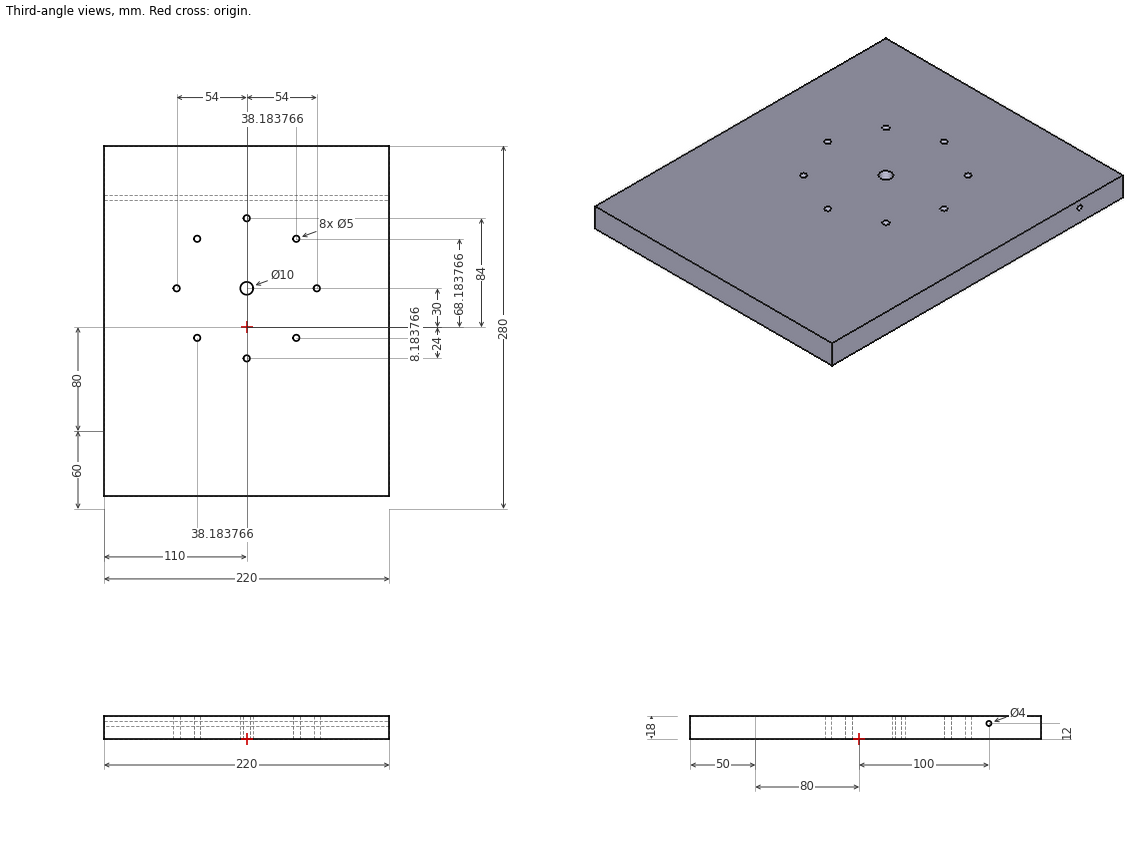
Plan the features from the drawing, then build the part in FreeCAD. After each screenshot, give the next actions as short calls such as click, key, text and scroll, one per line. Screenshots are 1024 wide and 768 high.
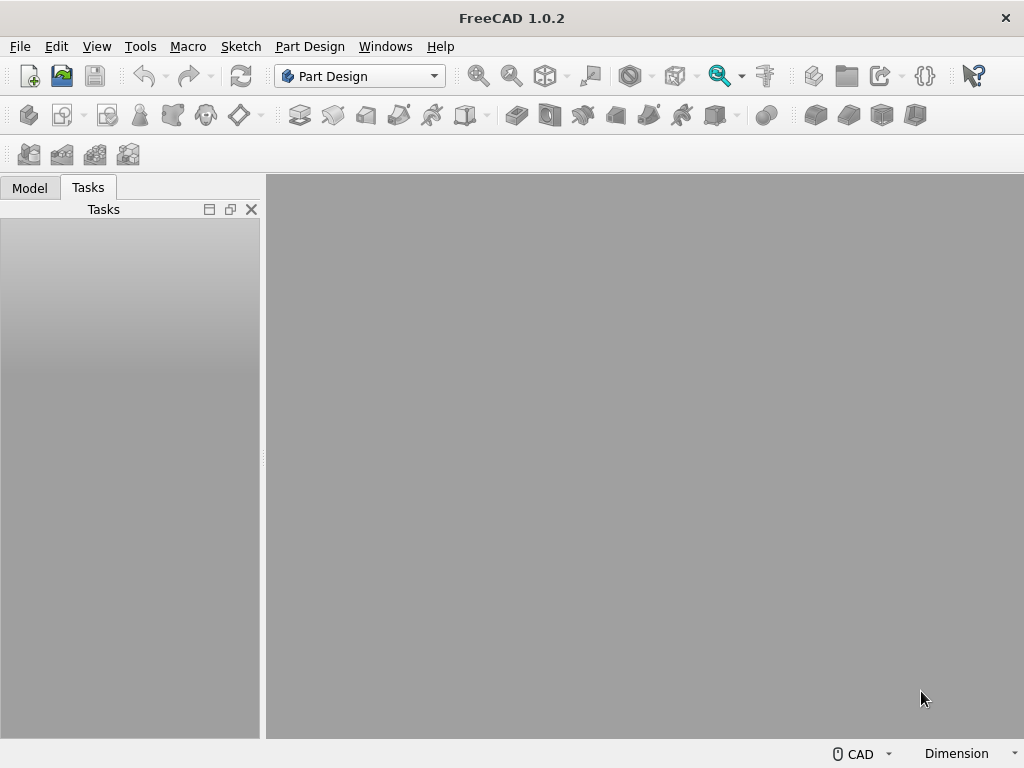
click(29, 76)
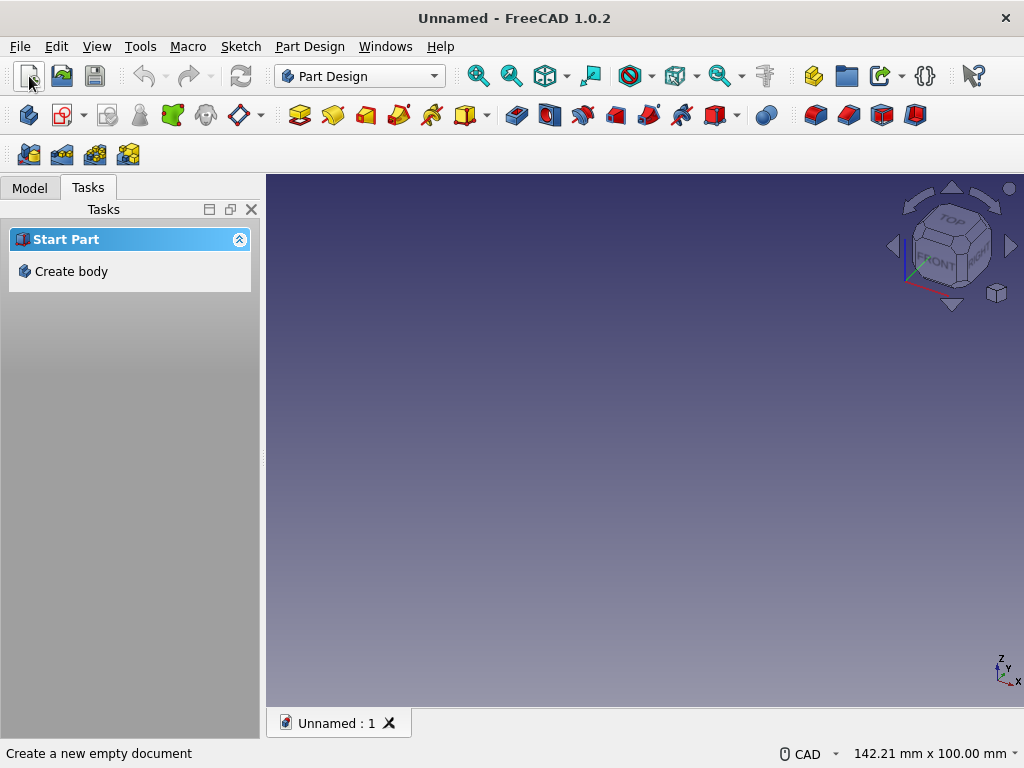
click(62, 116)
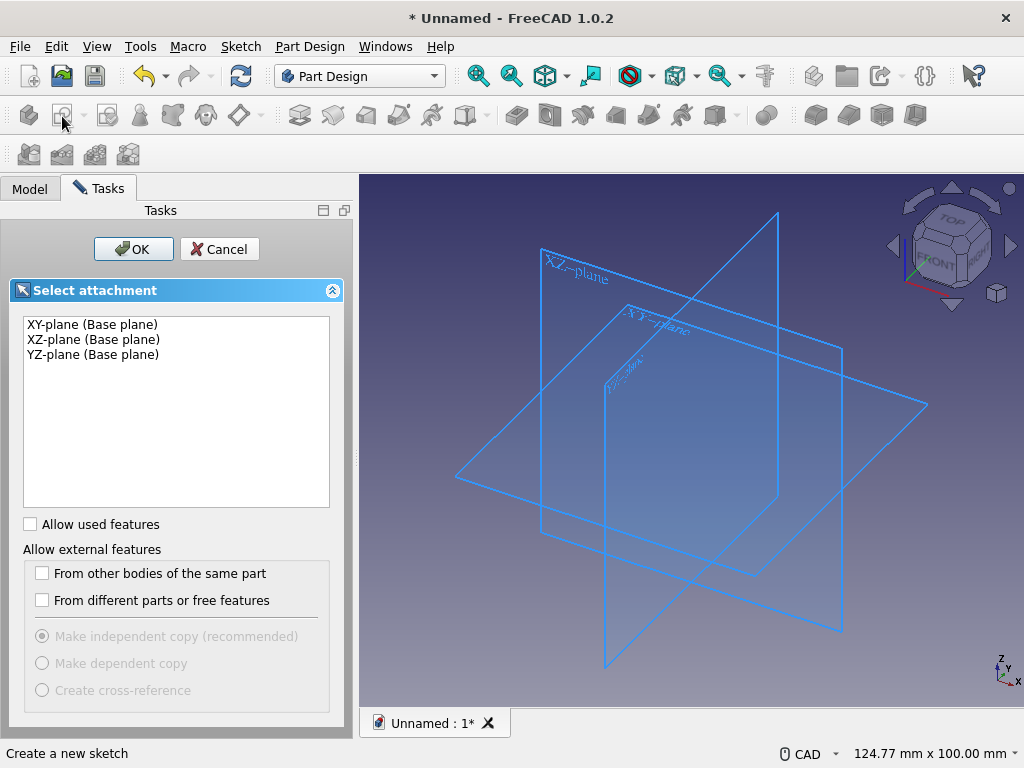
click(84, 324)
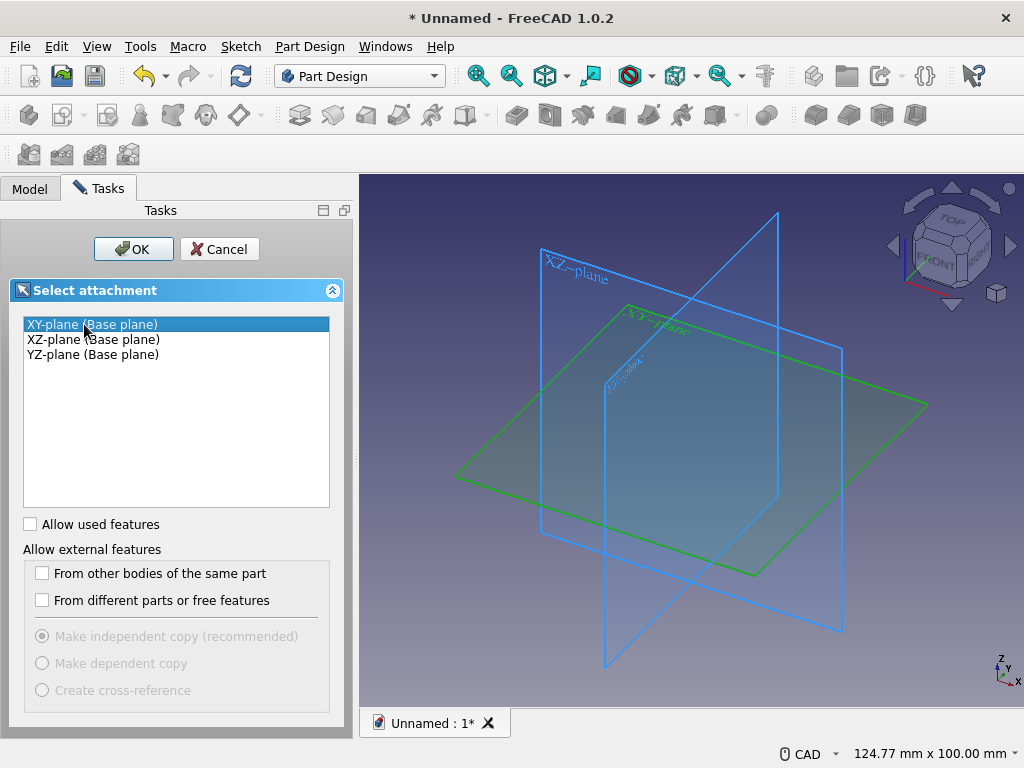
click(134, 249)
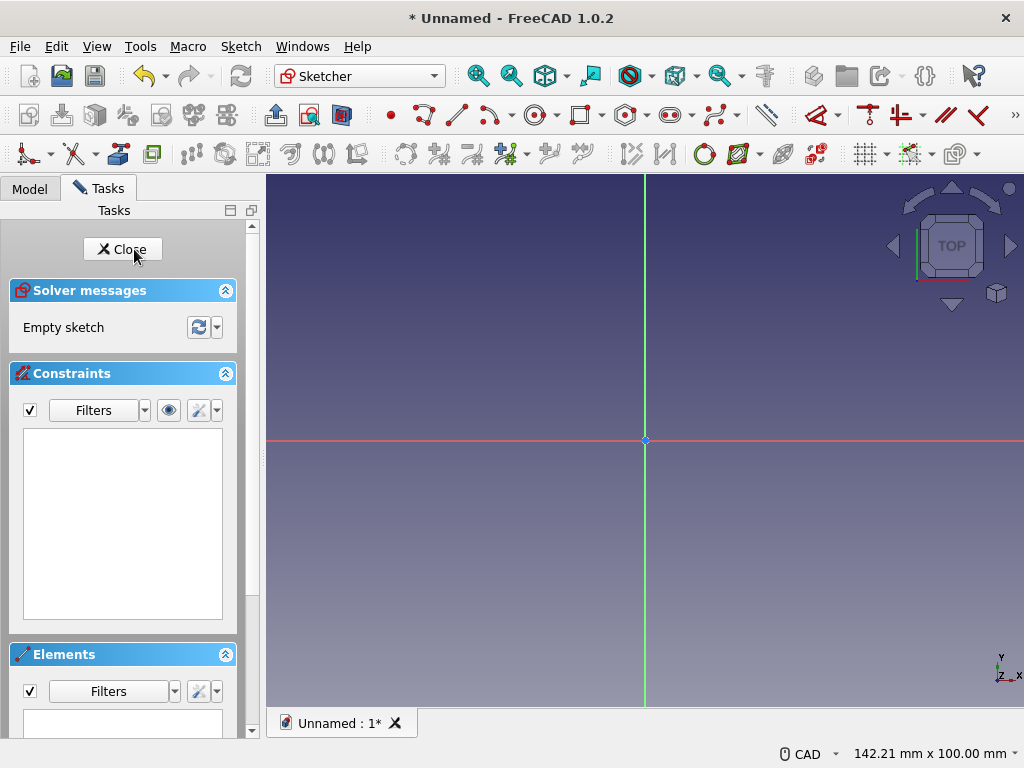
scroll(554, 440, down, 7)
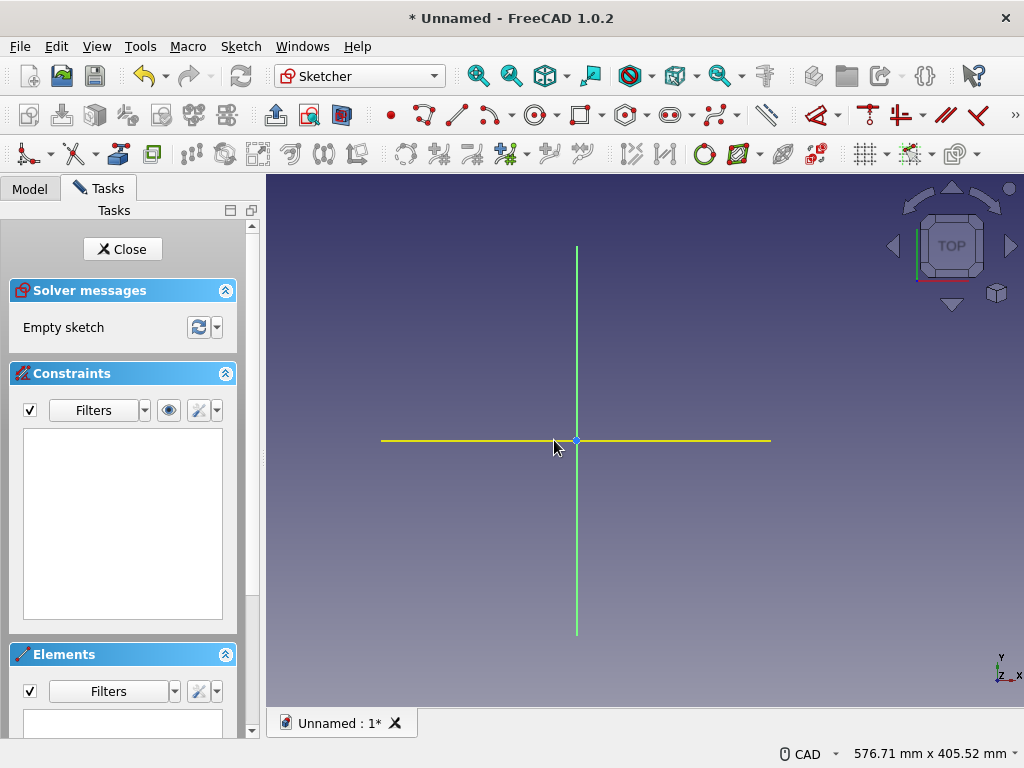
key(g)
key(v)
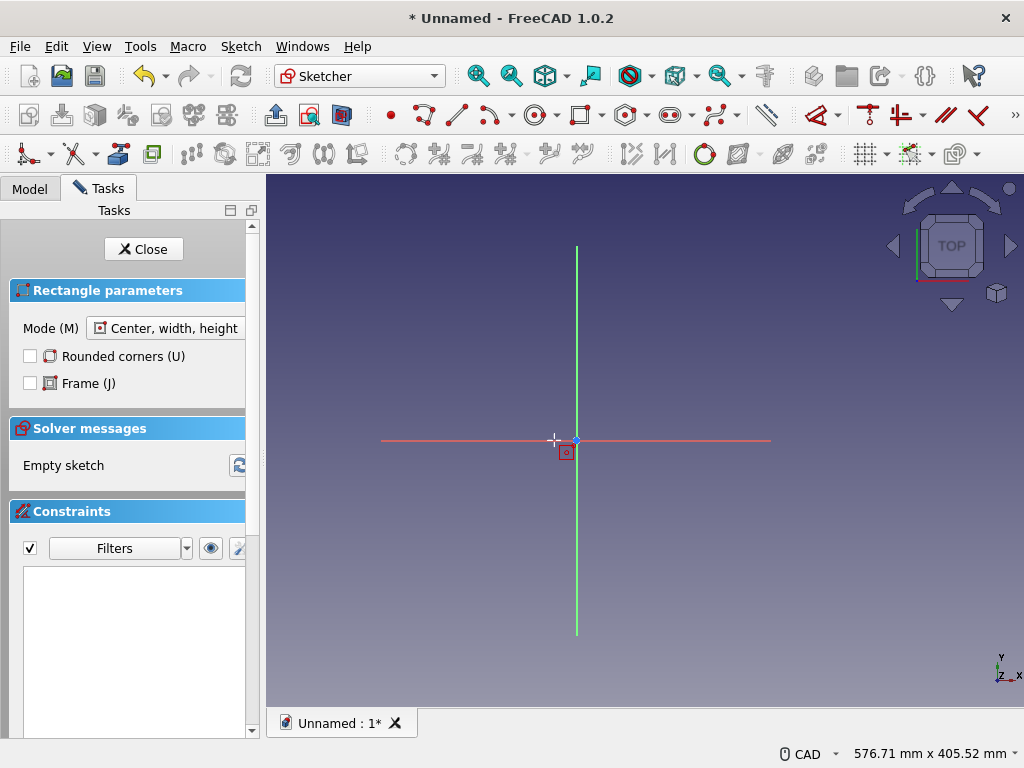
click(577, 440)
click(721, 256)
key(Escape)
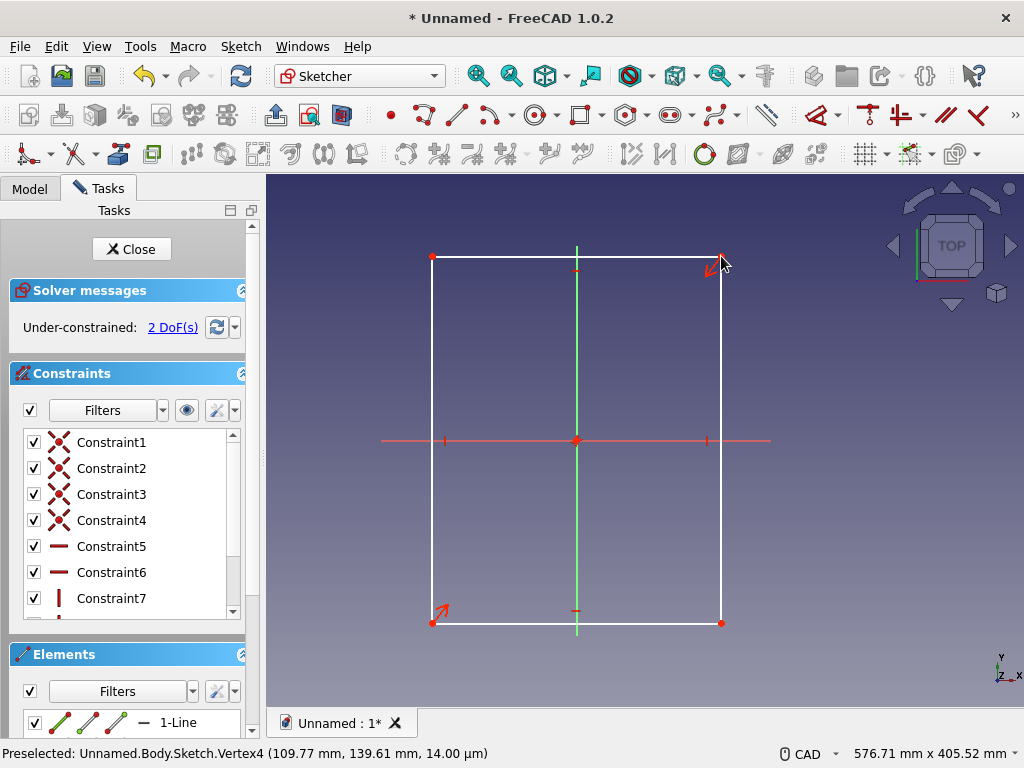
click(816, 116)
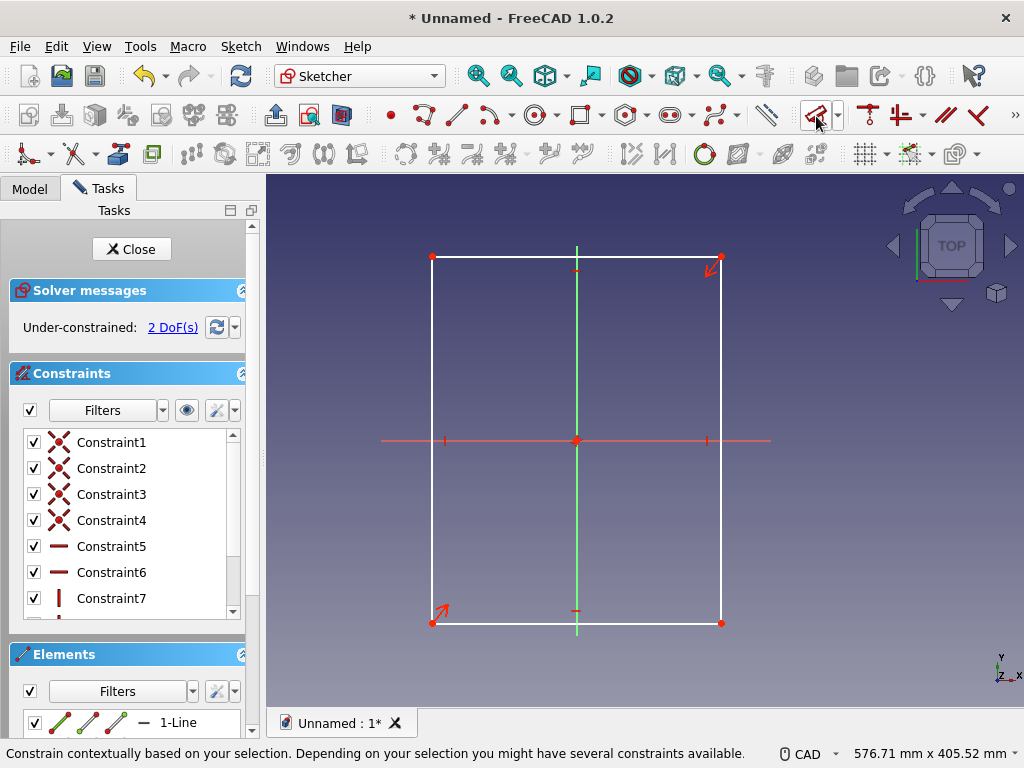
click(519, 624)
click(510, 658)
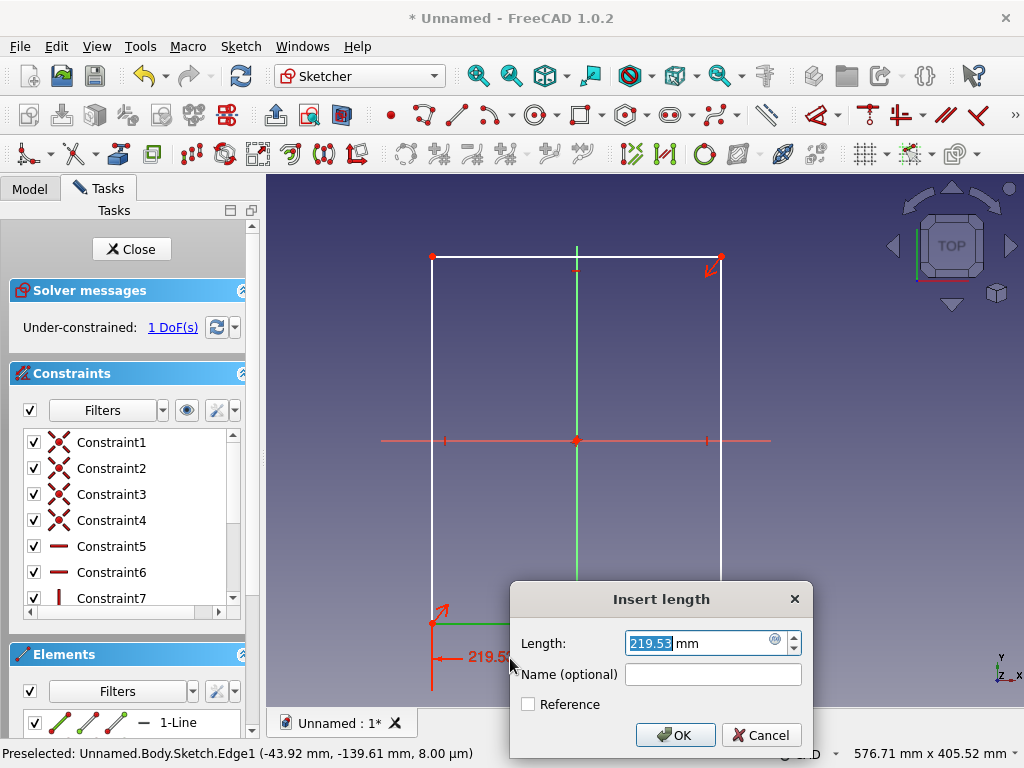
text(220)
key(Return)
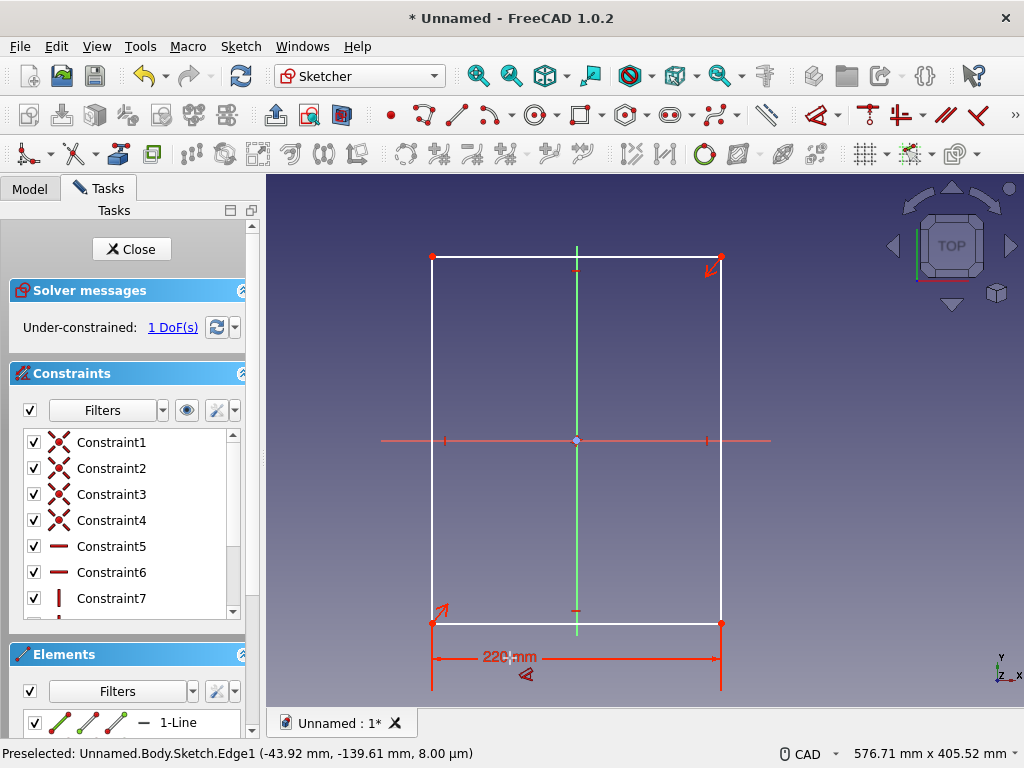
click(721, 514)
click(755, 356)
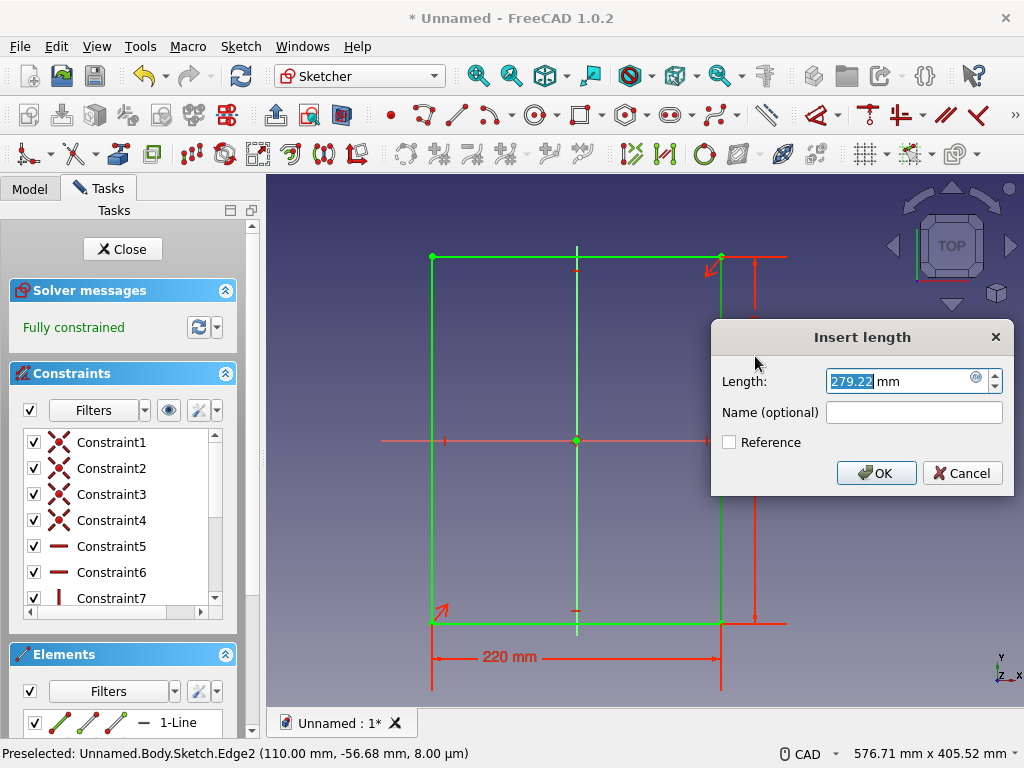
text(280)
key(Return)
key(Escape)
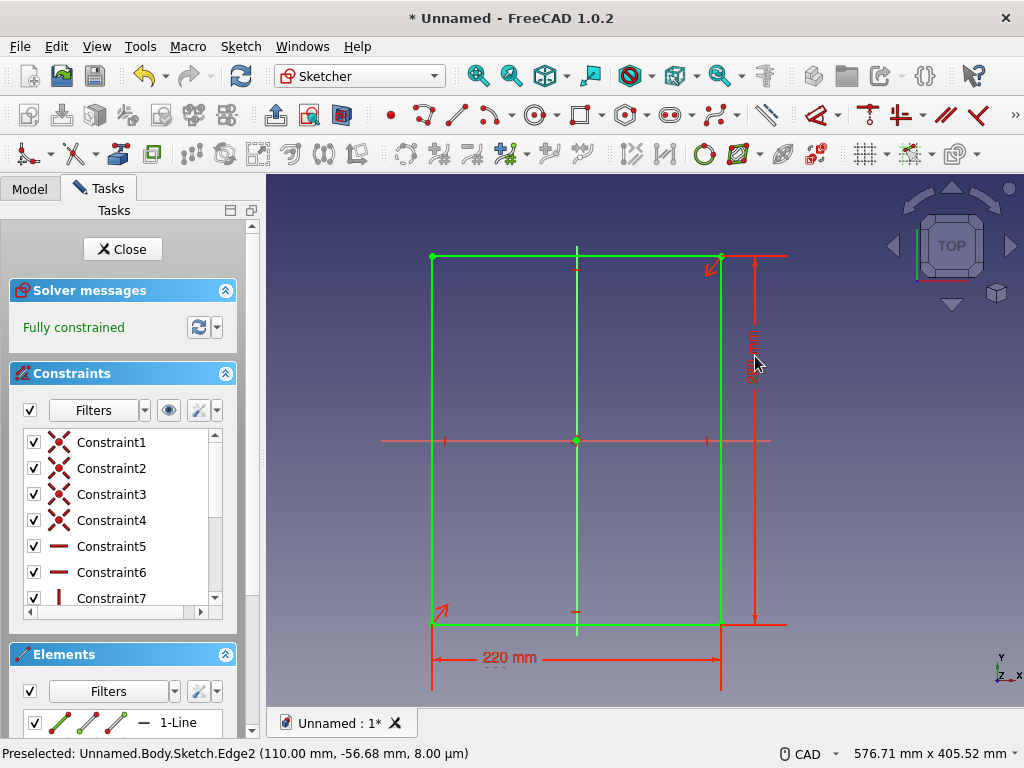
click(123, 249)